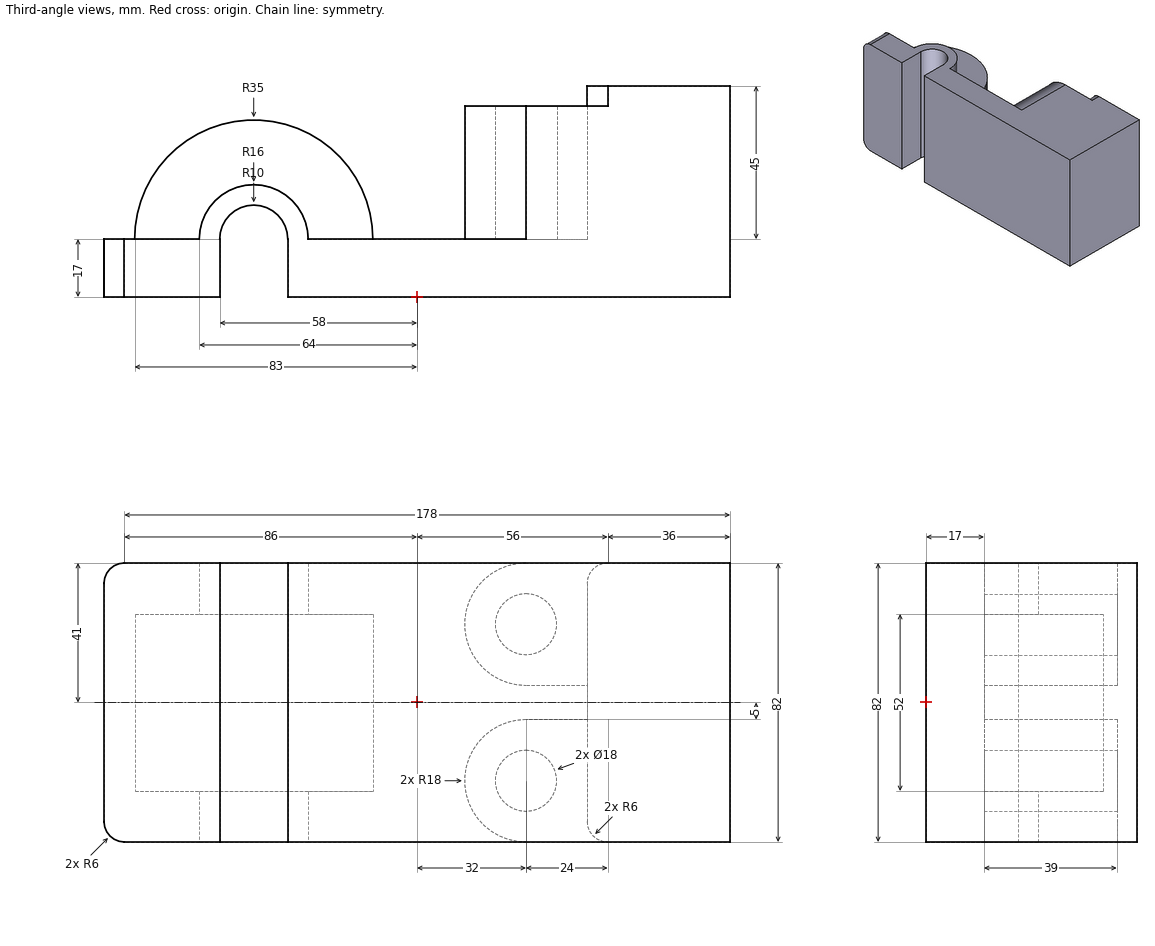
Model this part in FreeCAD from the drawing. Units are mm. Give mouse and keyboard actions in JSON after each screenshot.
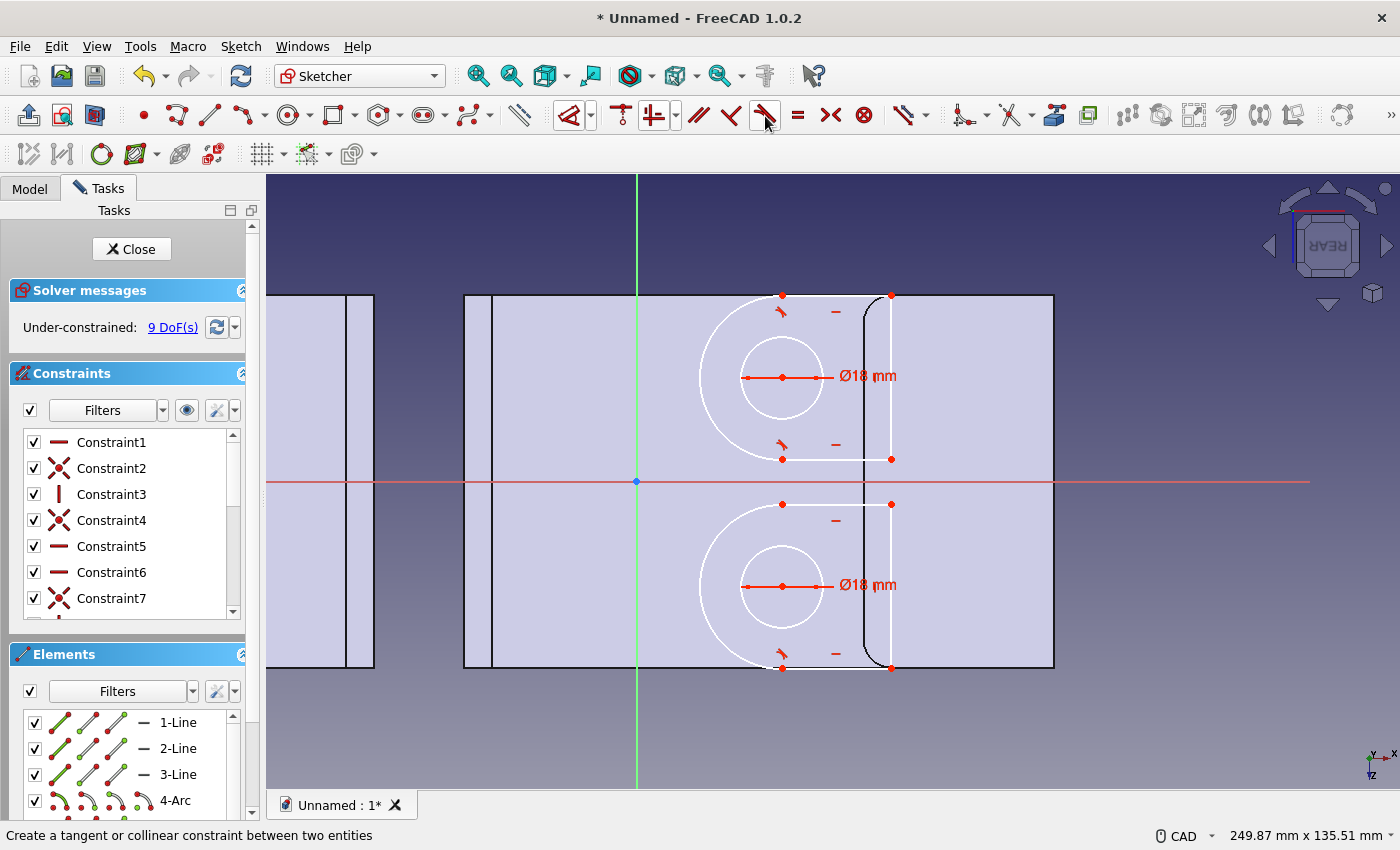
{"action": "left_click", "coordinate": [858, 505]}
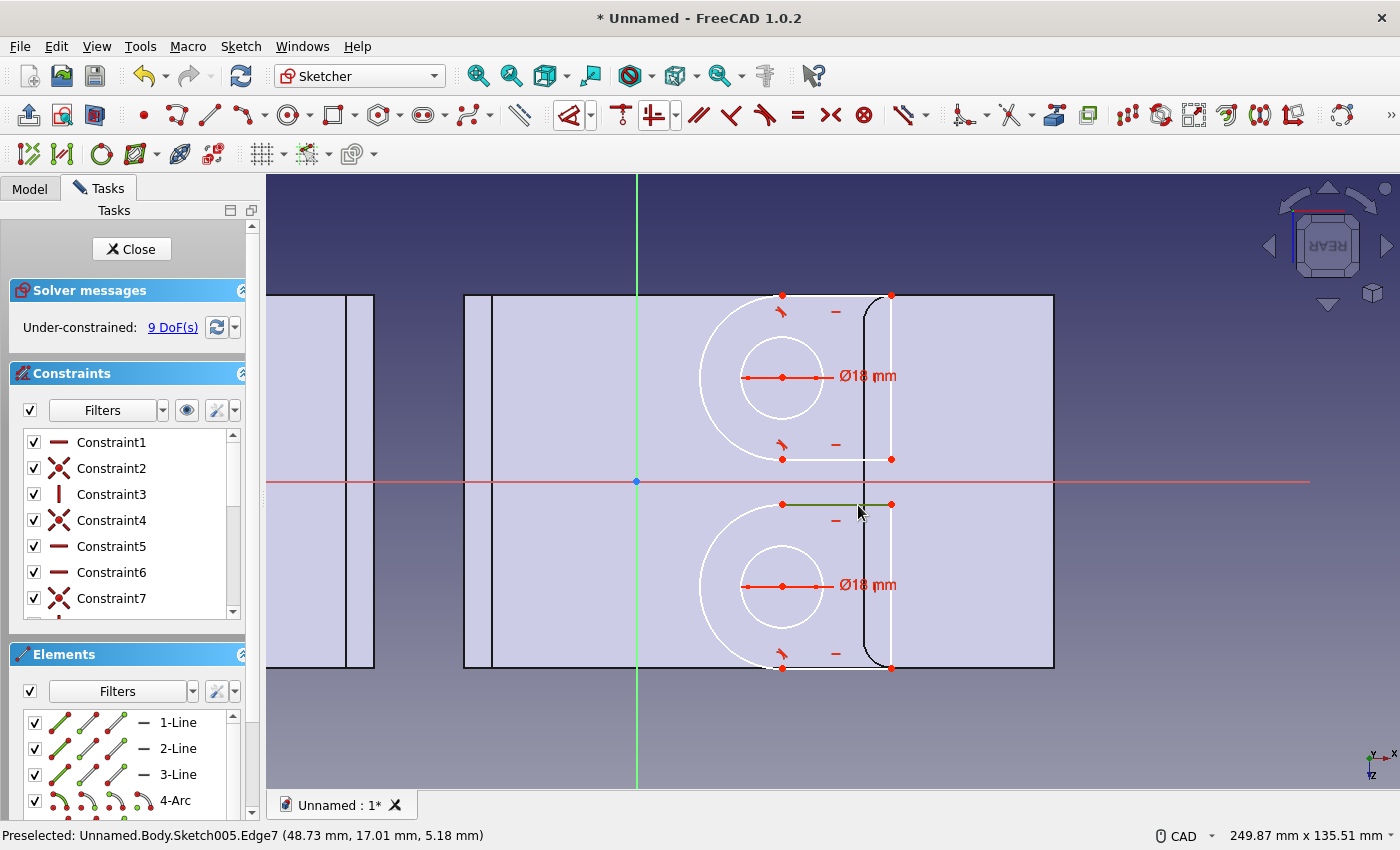
{"action": "left_click", "coordinate": [716, 539]}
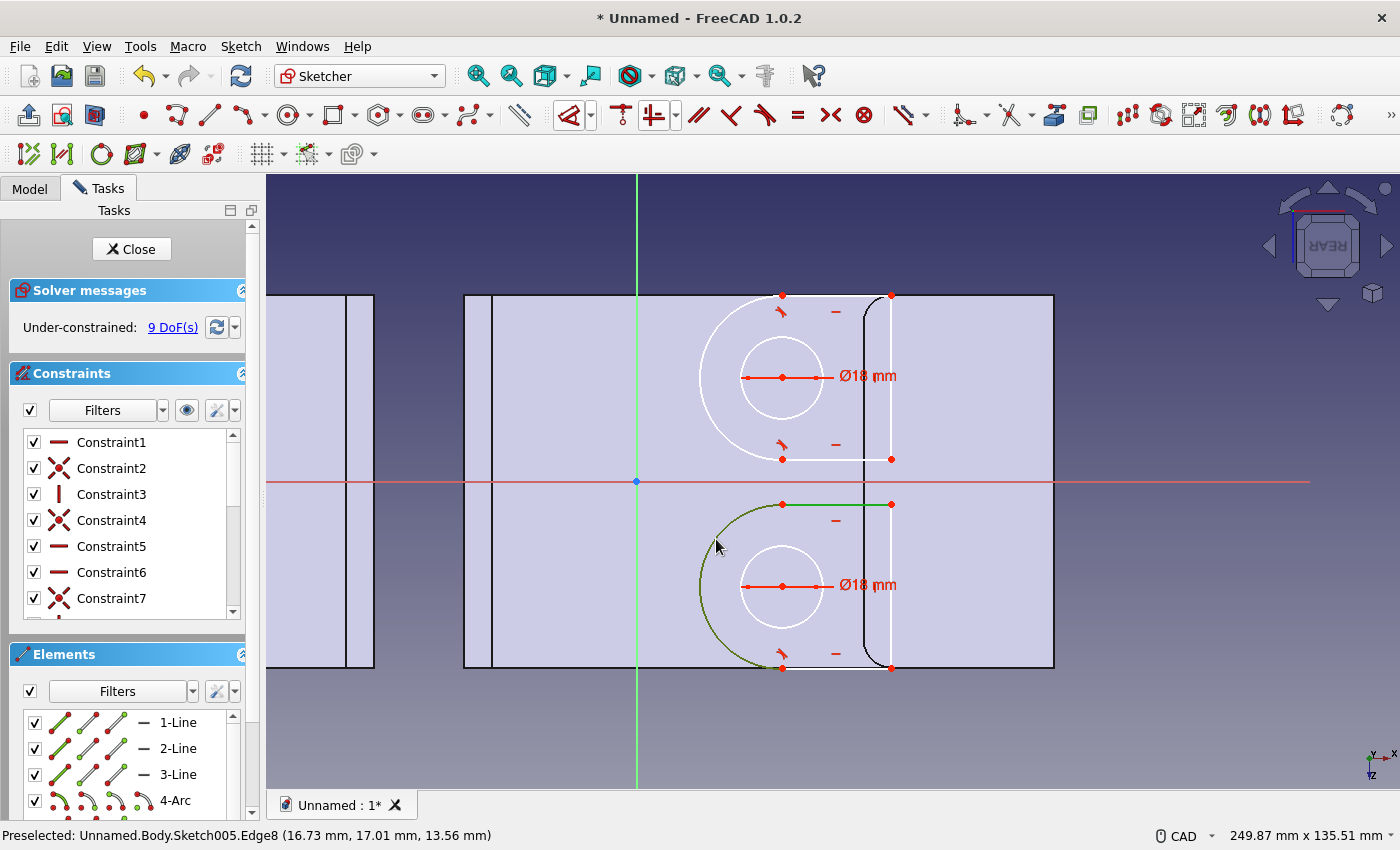
{"action": "left_click", "coordinate": [765, 116]}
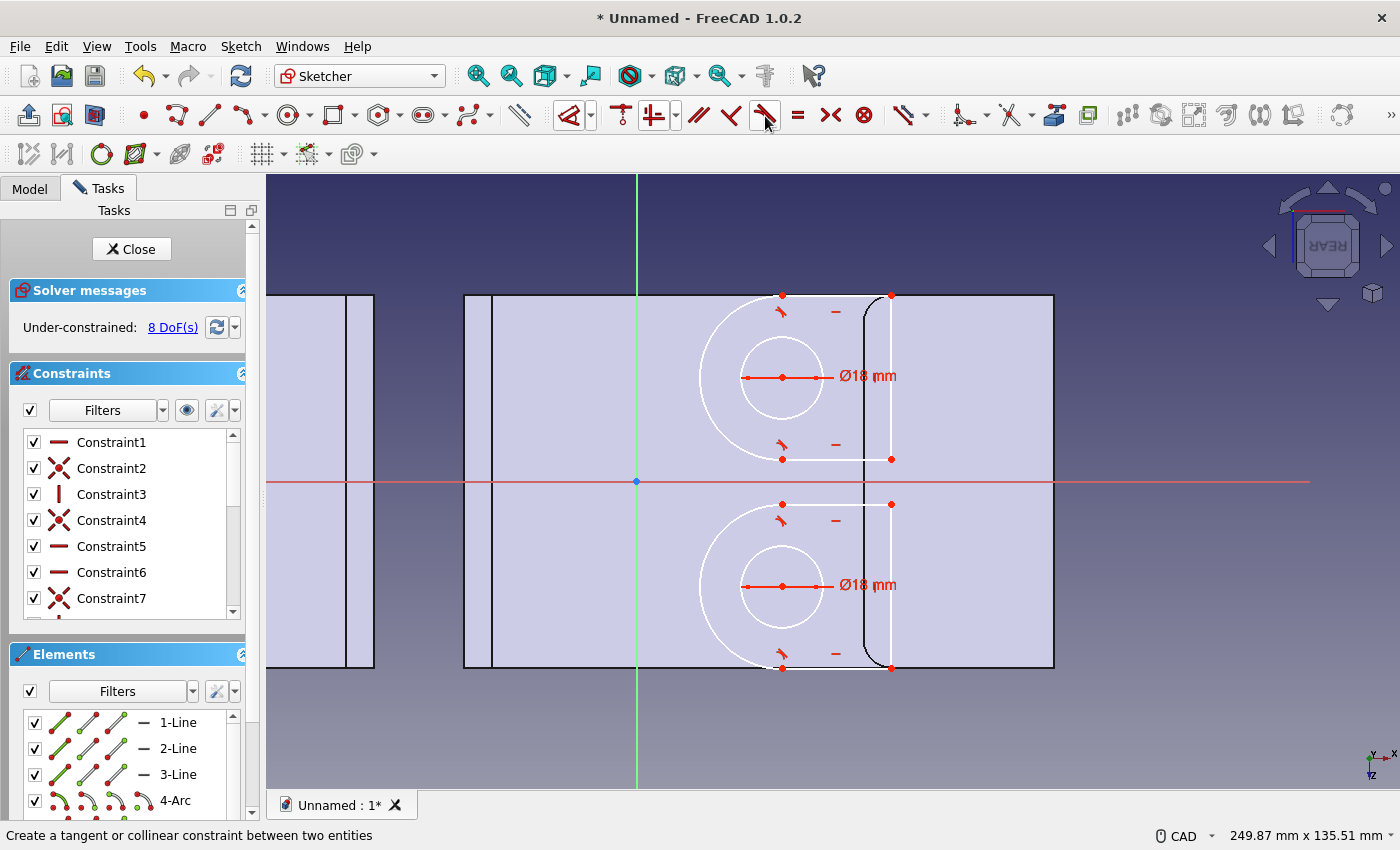
{"action": "left_click", "coordinate": [716, 330]}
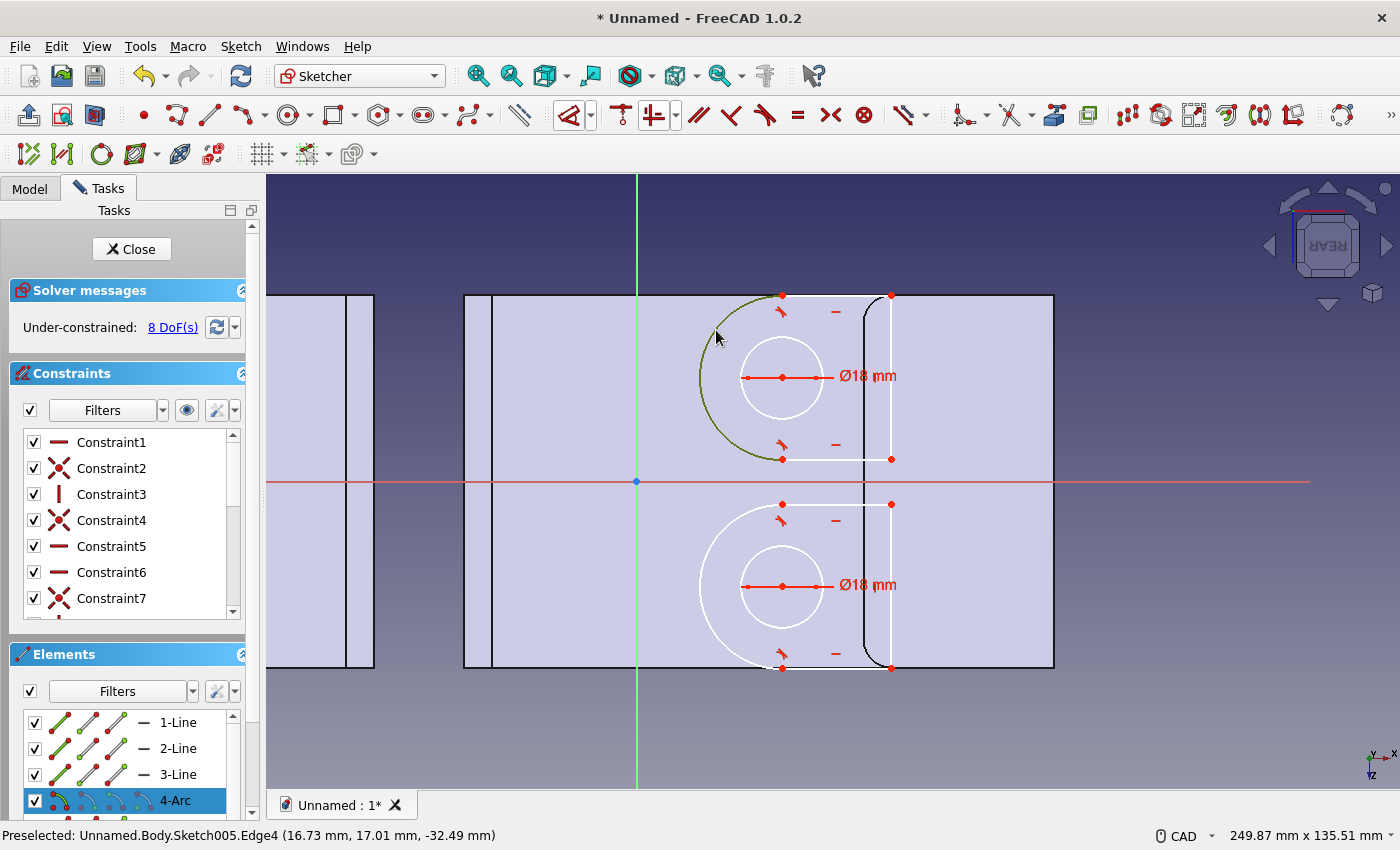
{"action": "left_click", "coordinate": [716, 539]}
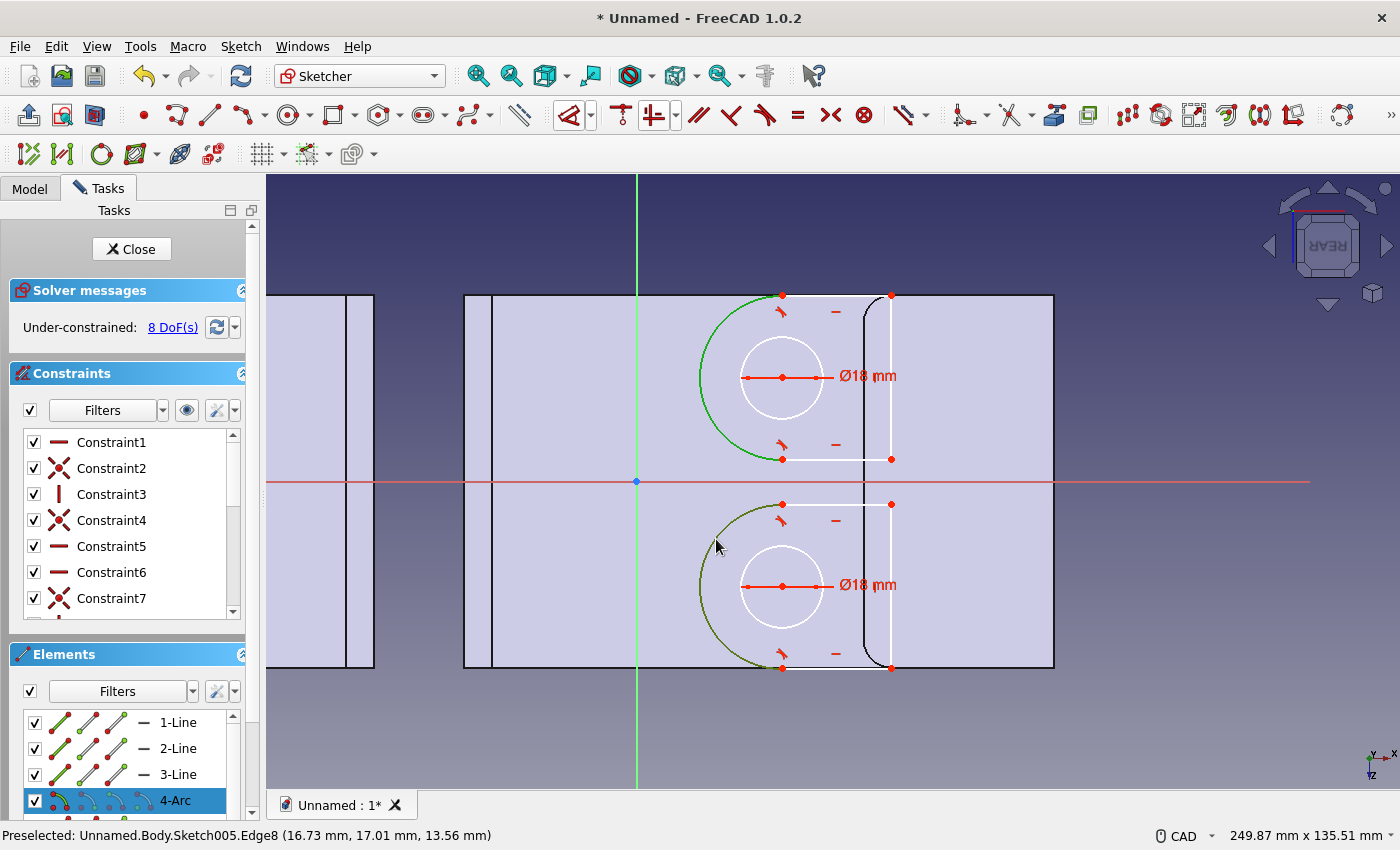
{"action": "left_click", "coordinate": [798, 116]}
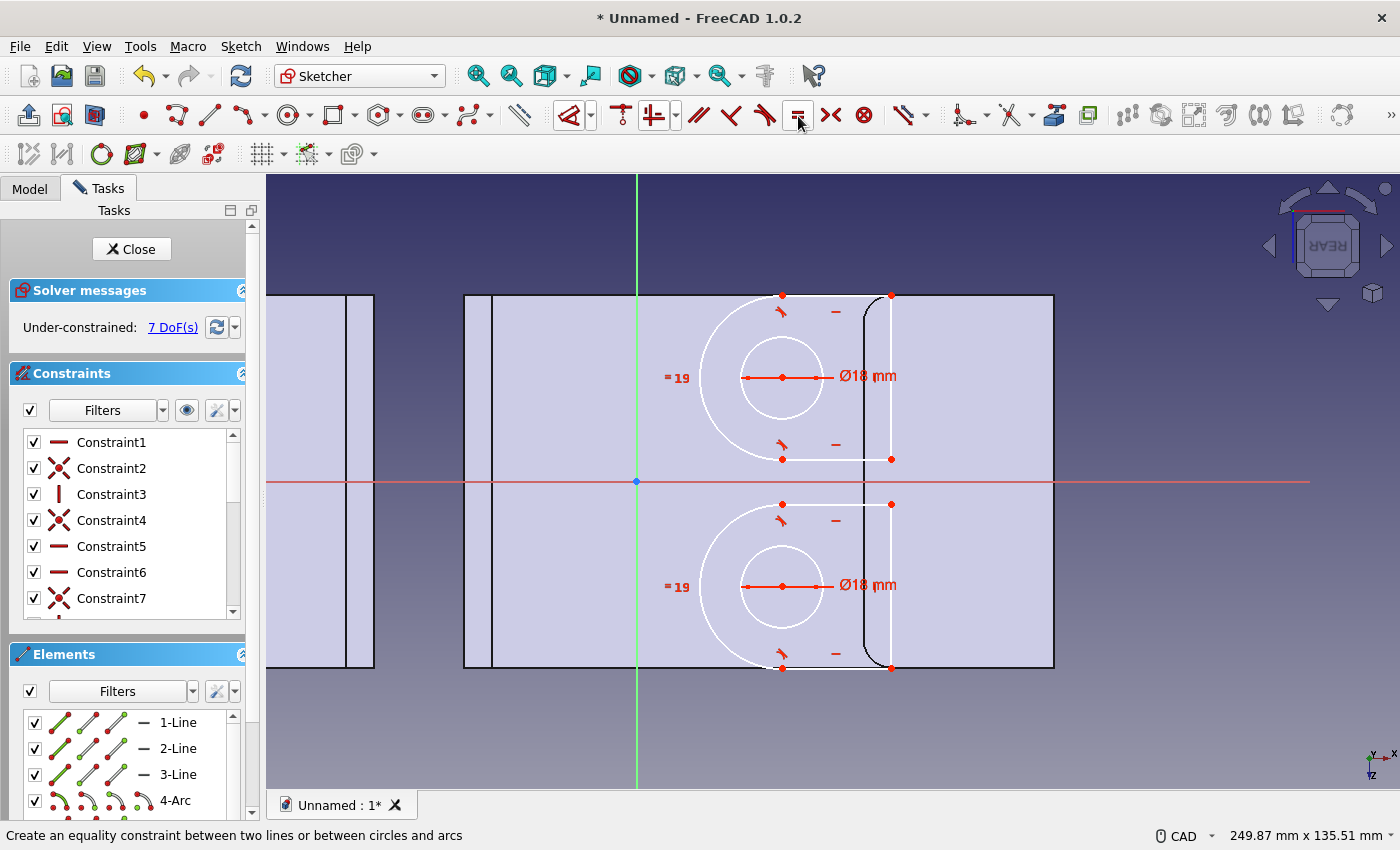
{"action": "left_click", "coordinate": [782, 378]}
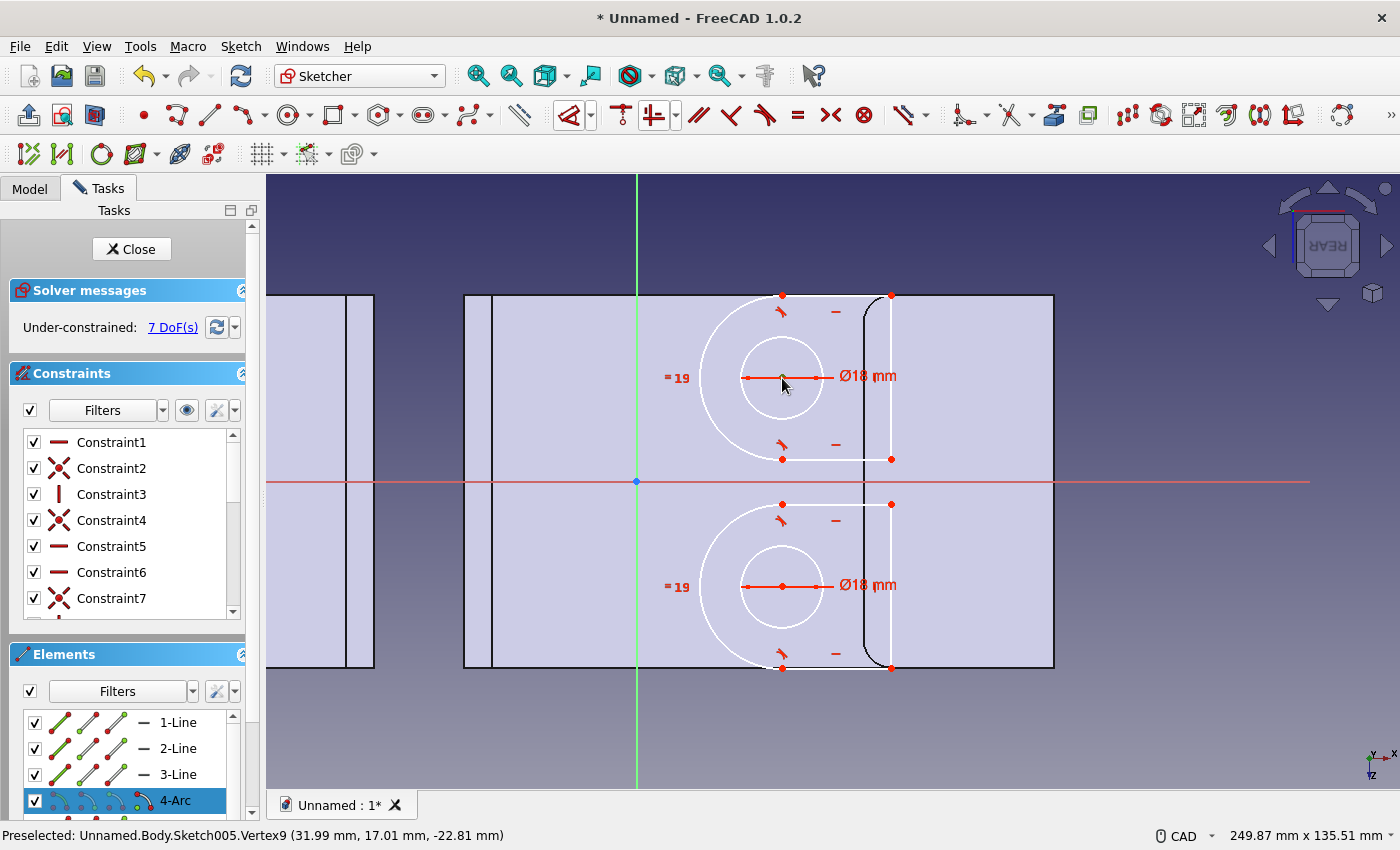
{"action": "left_click", "coordinate": [782, 587]}